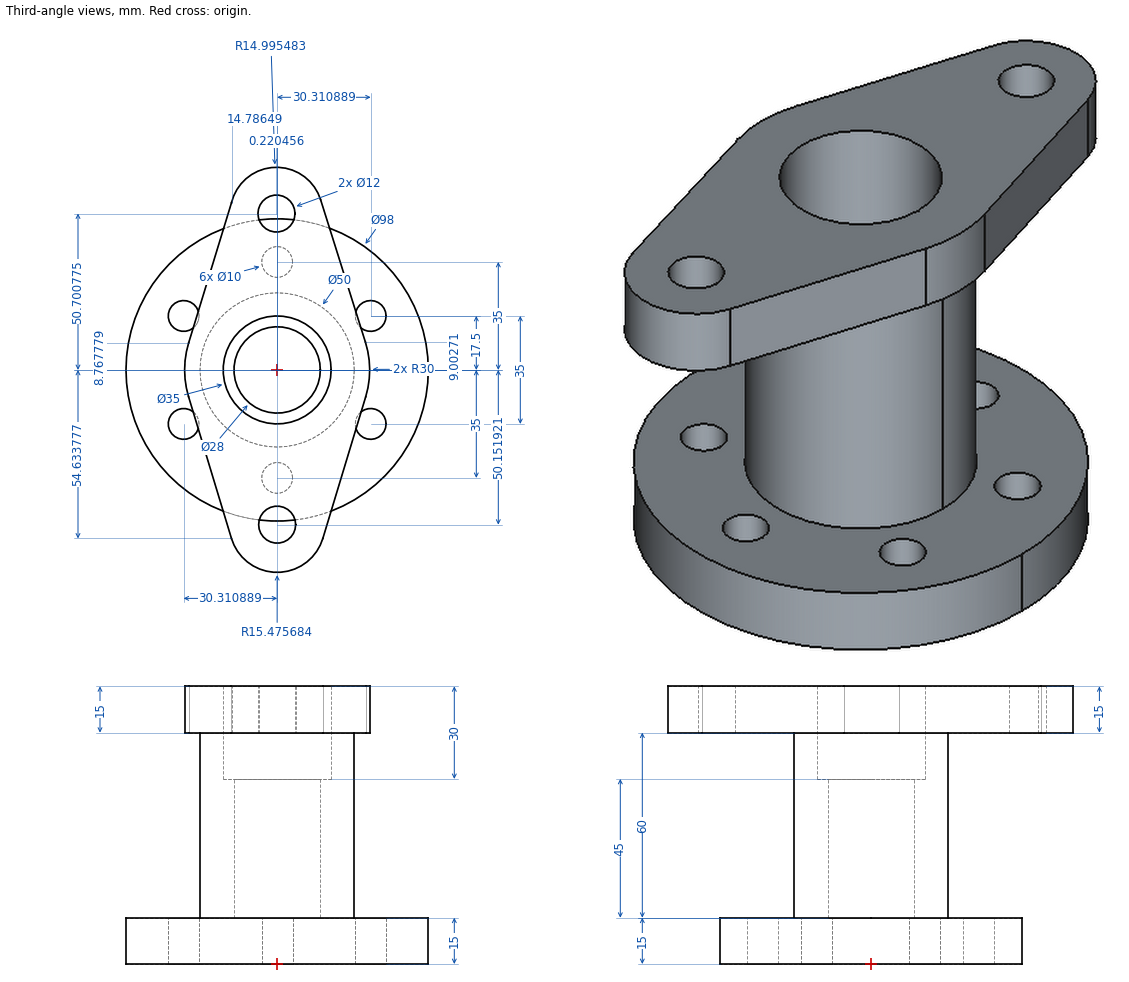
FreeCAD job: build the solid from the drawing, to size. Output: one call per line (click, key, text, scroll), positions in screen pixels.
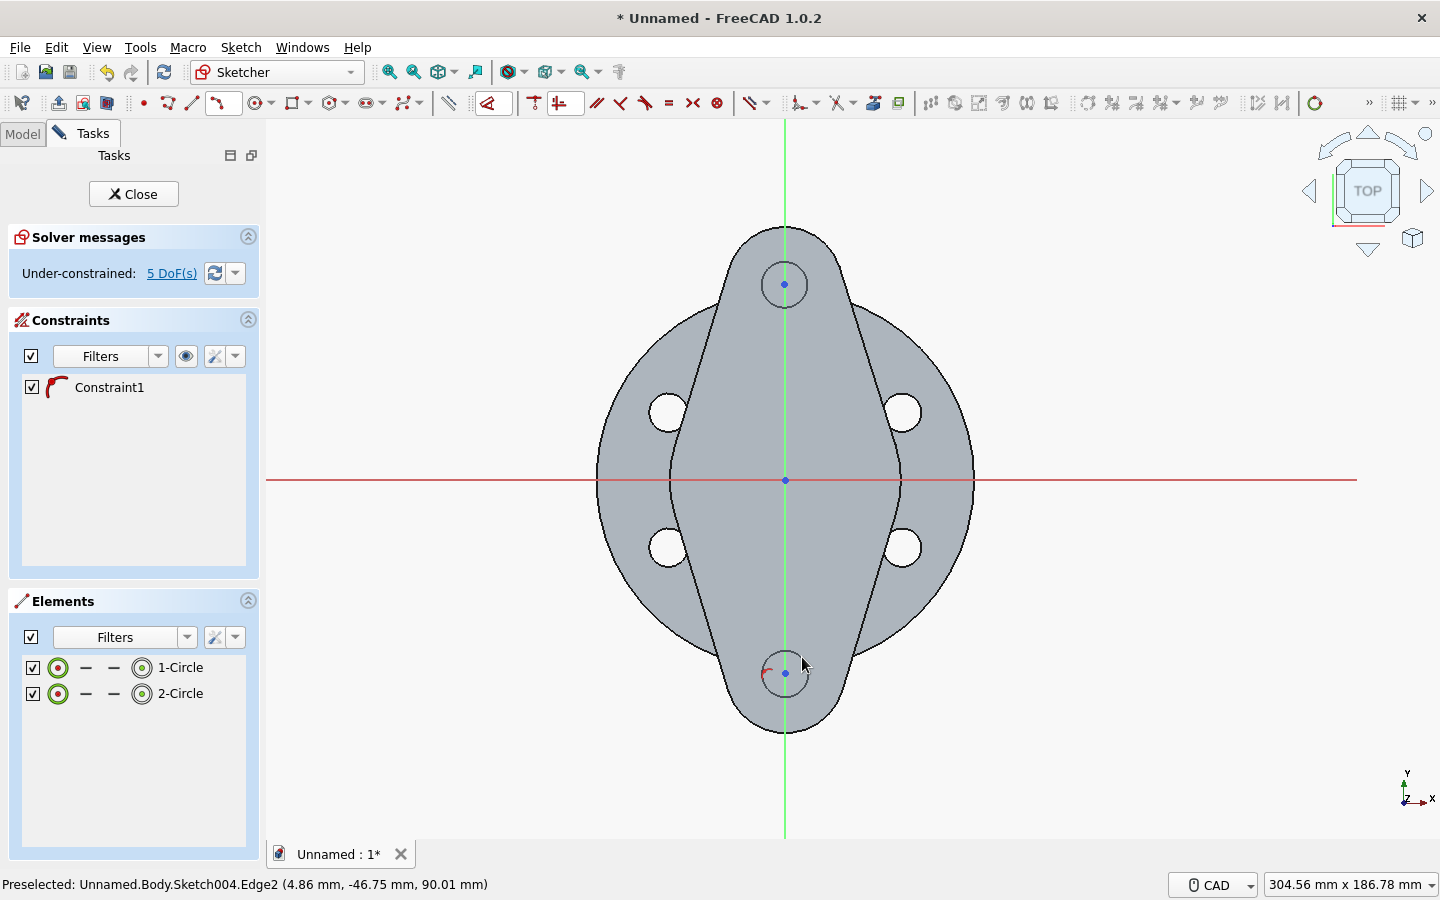
click(801, 269)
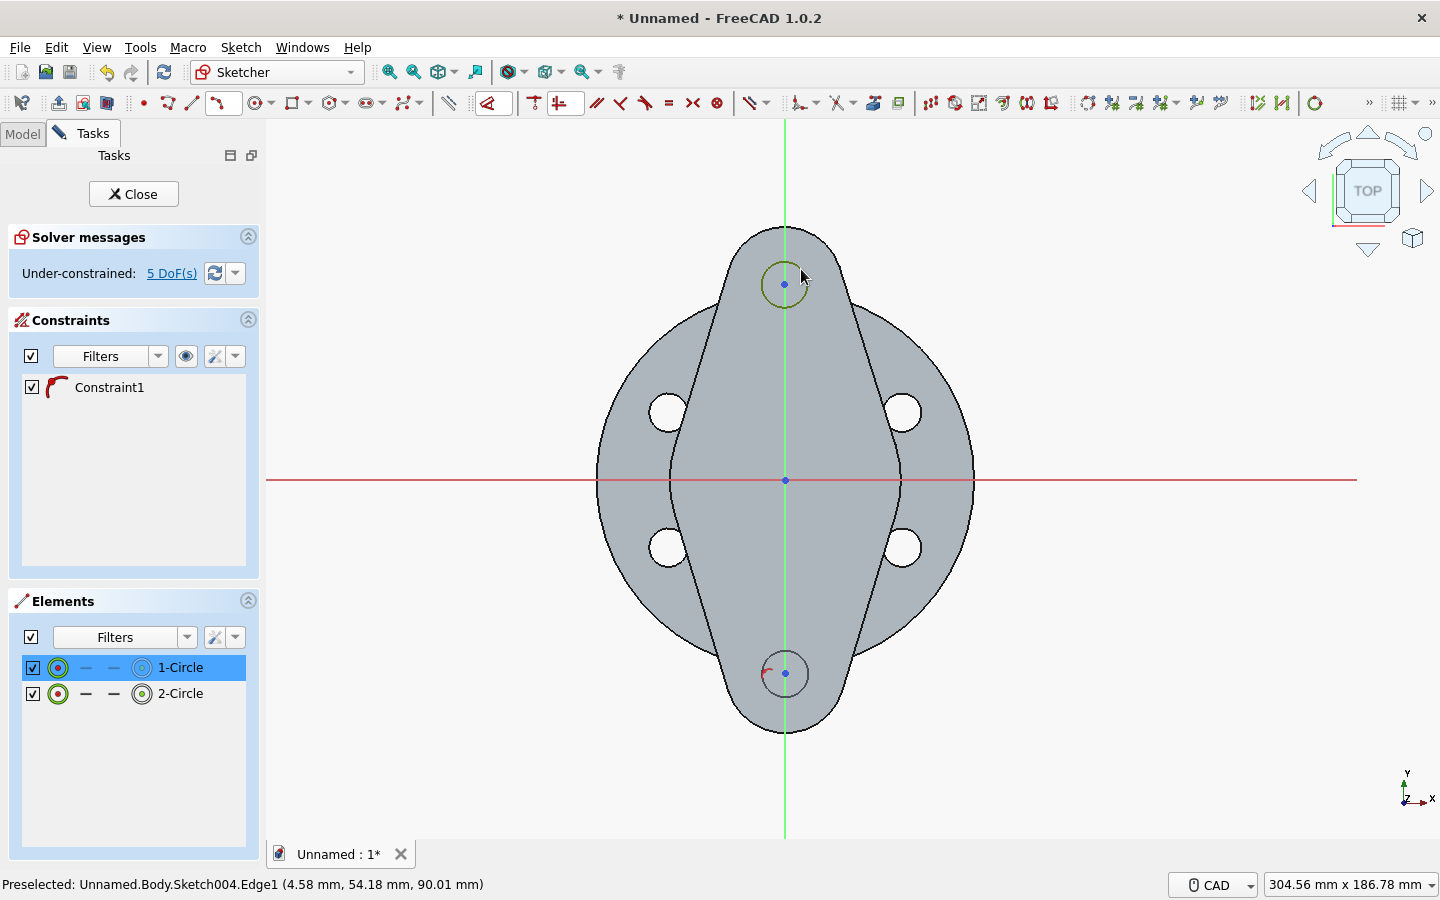
click(802, 658)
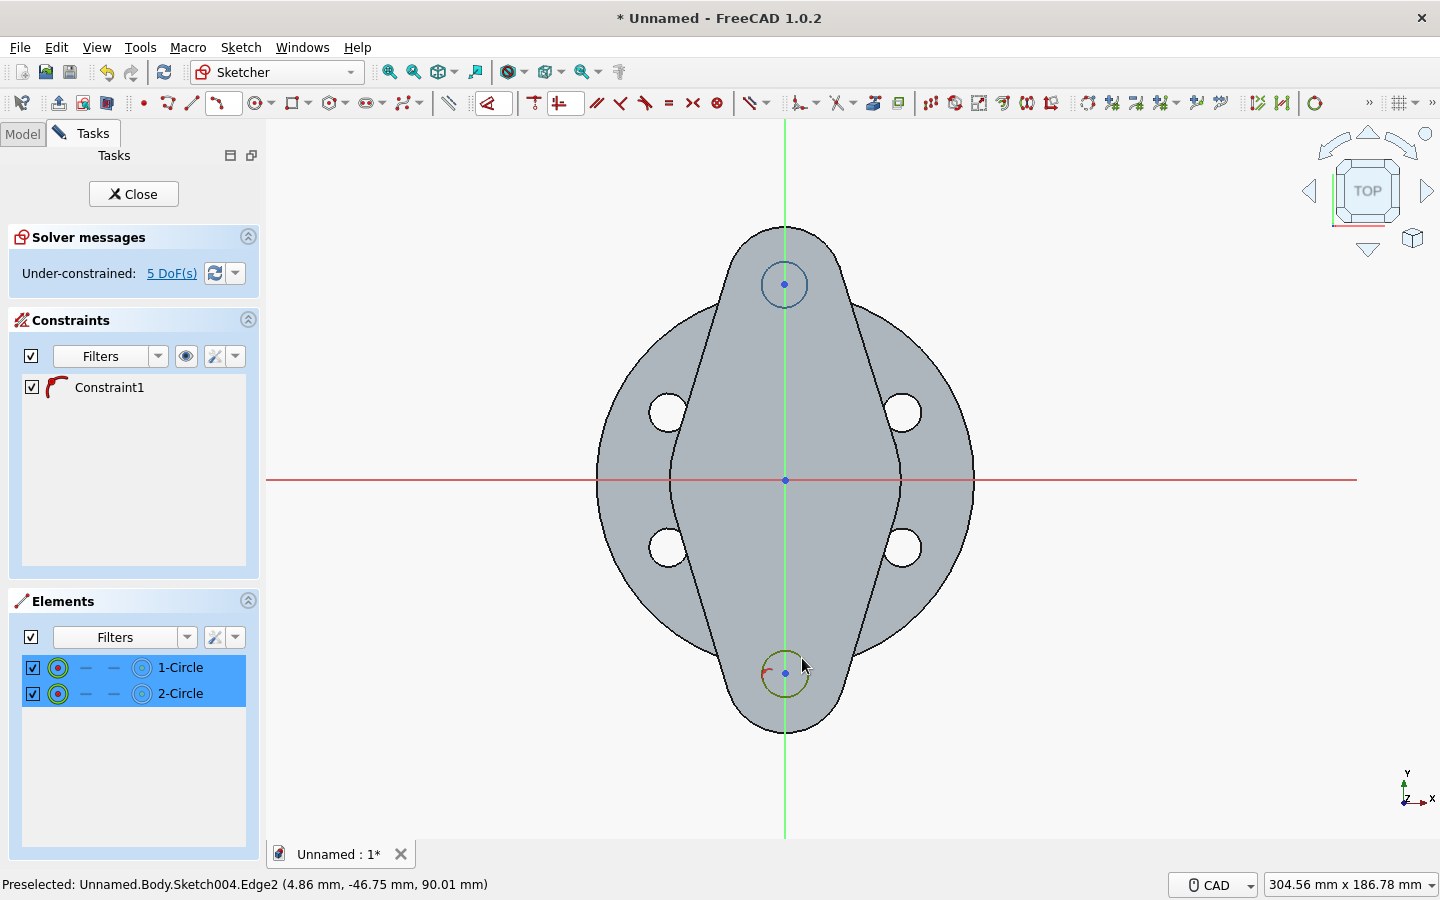
key(e)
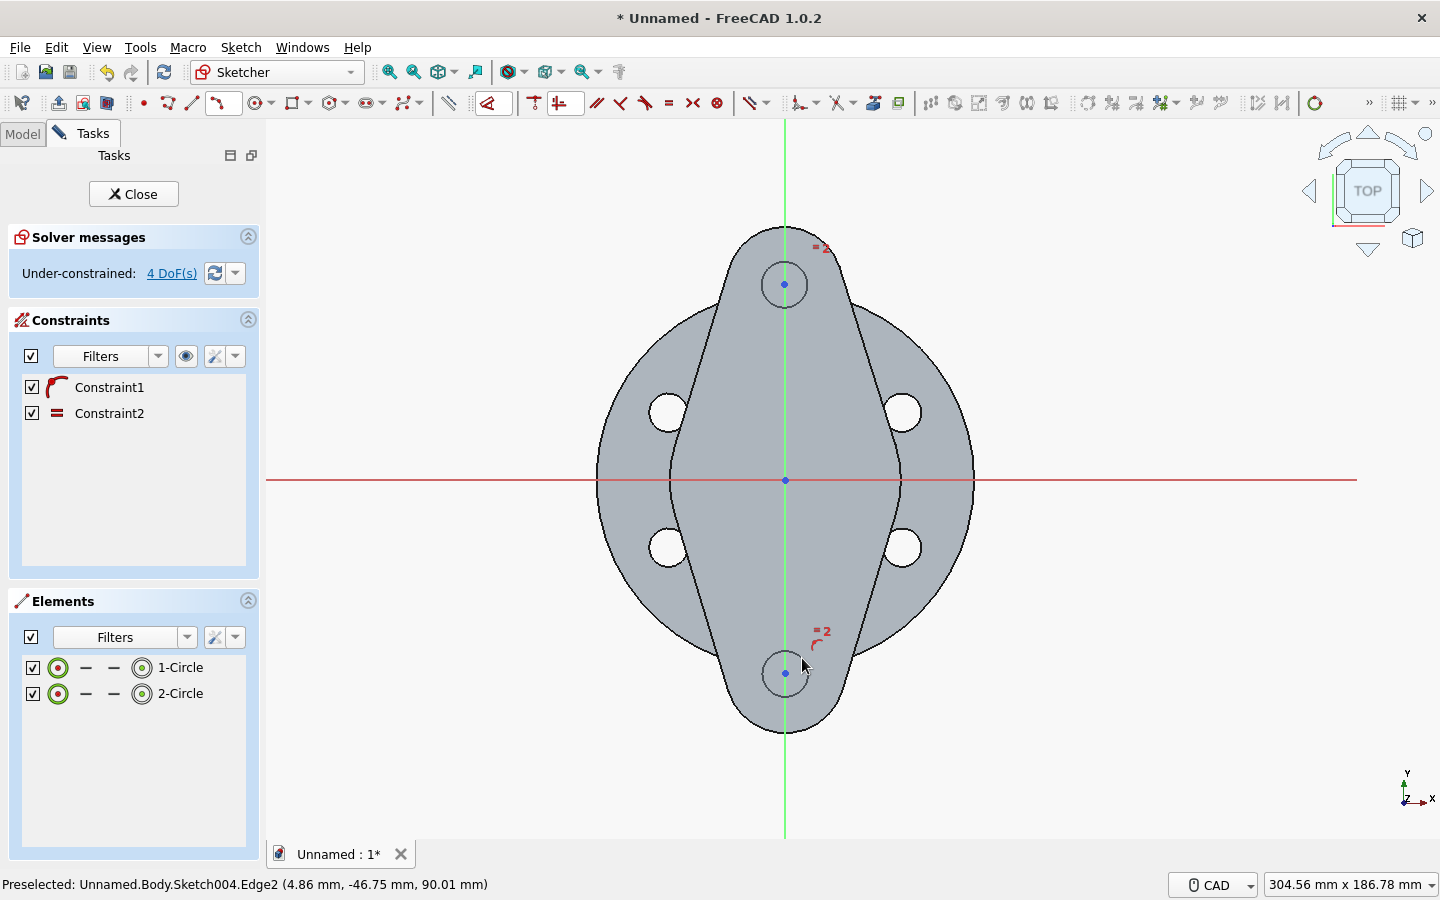
click(801, 269)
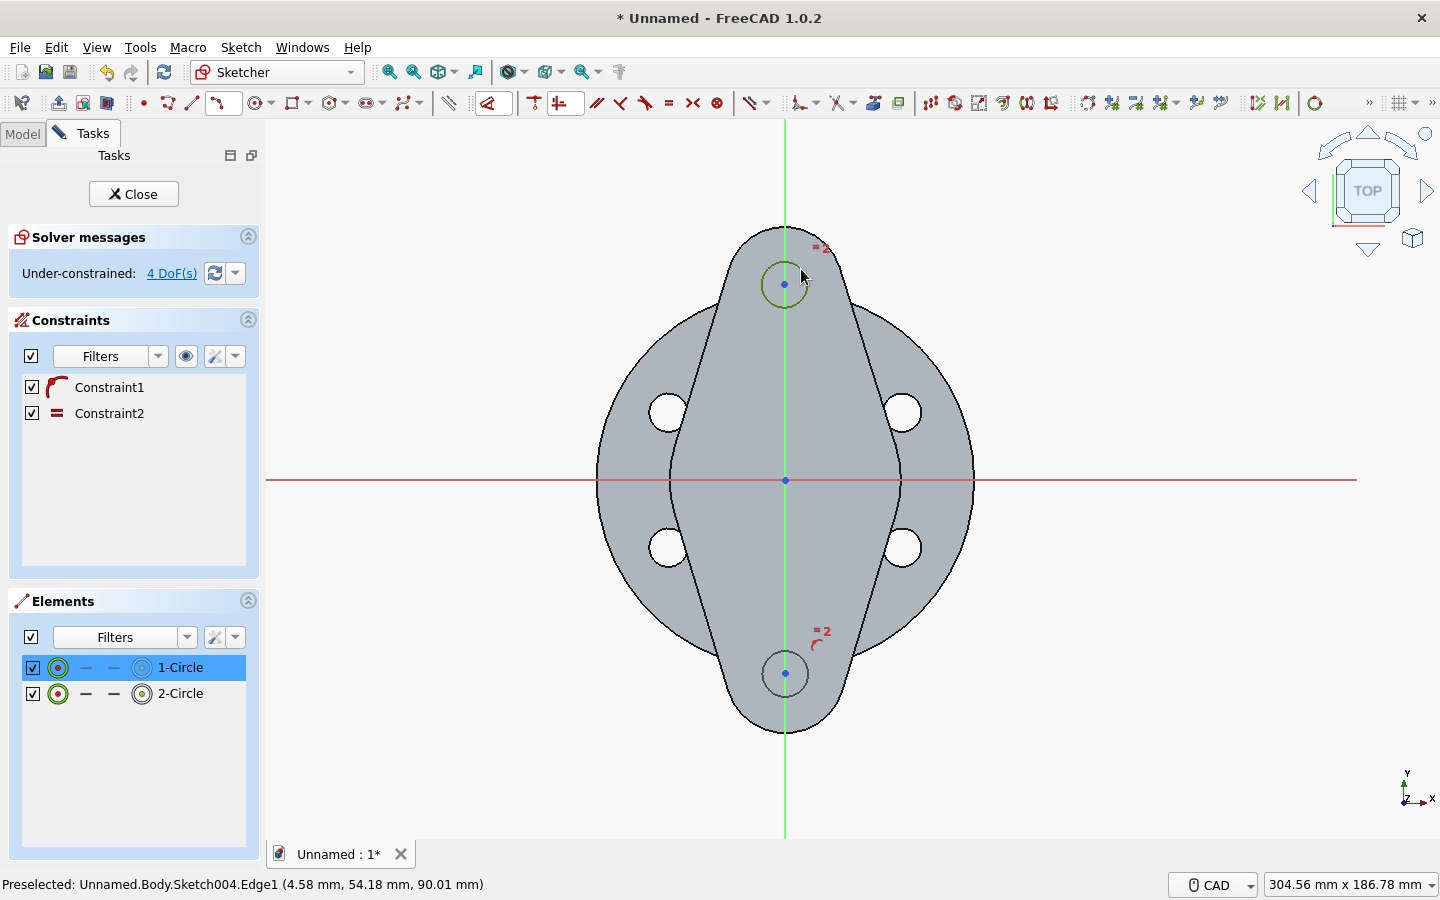
click(506, 104)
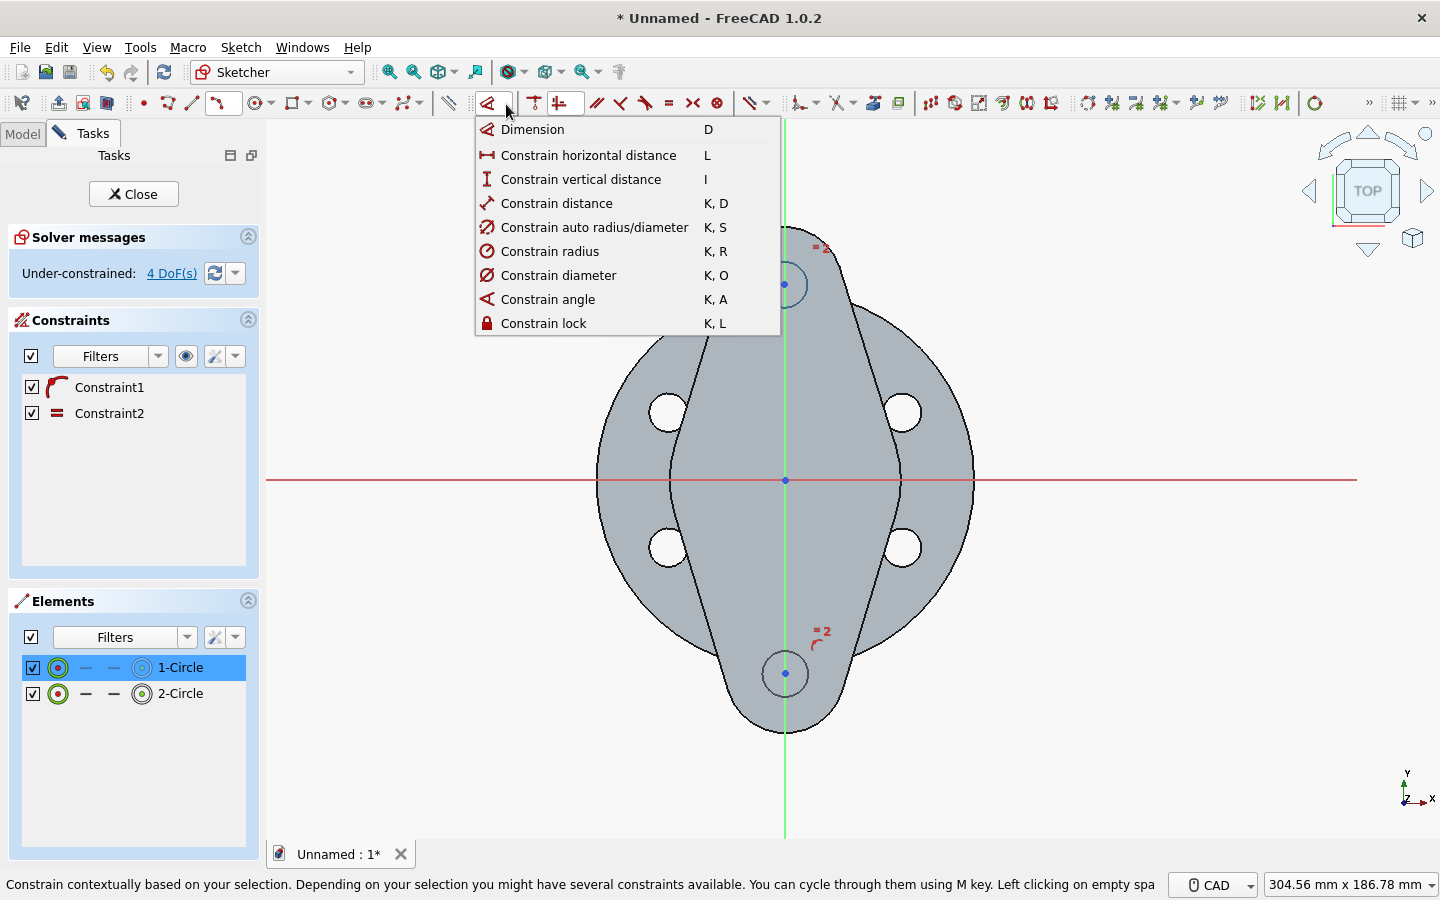
click(628, 275)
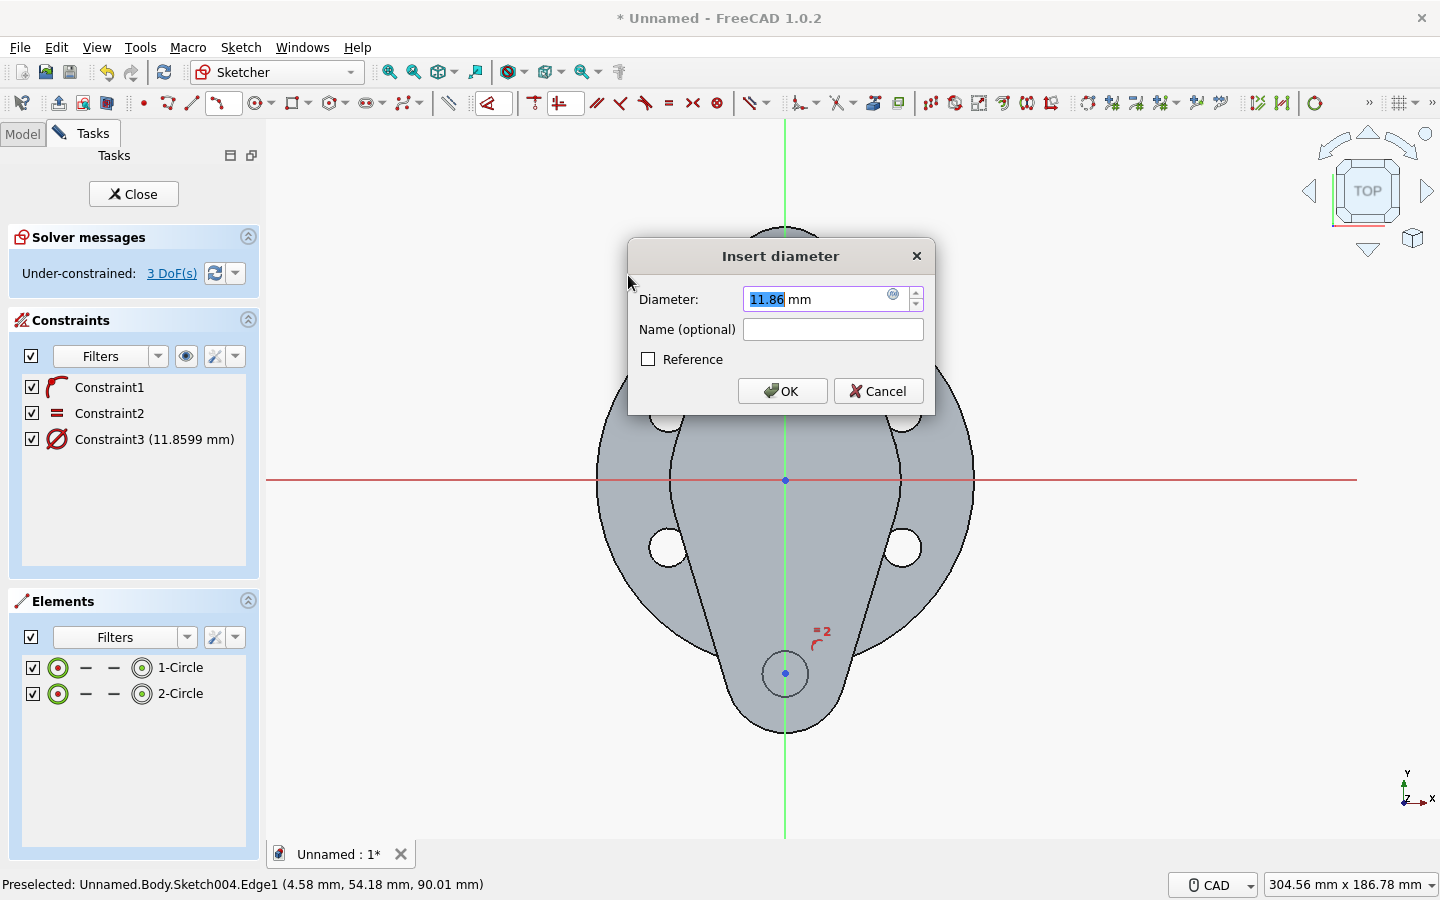
text(12)
key(Return)